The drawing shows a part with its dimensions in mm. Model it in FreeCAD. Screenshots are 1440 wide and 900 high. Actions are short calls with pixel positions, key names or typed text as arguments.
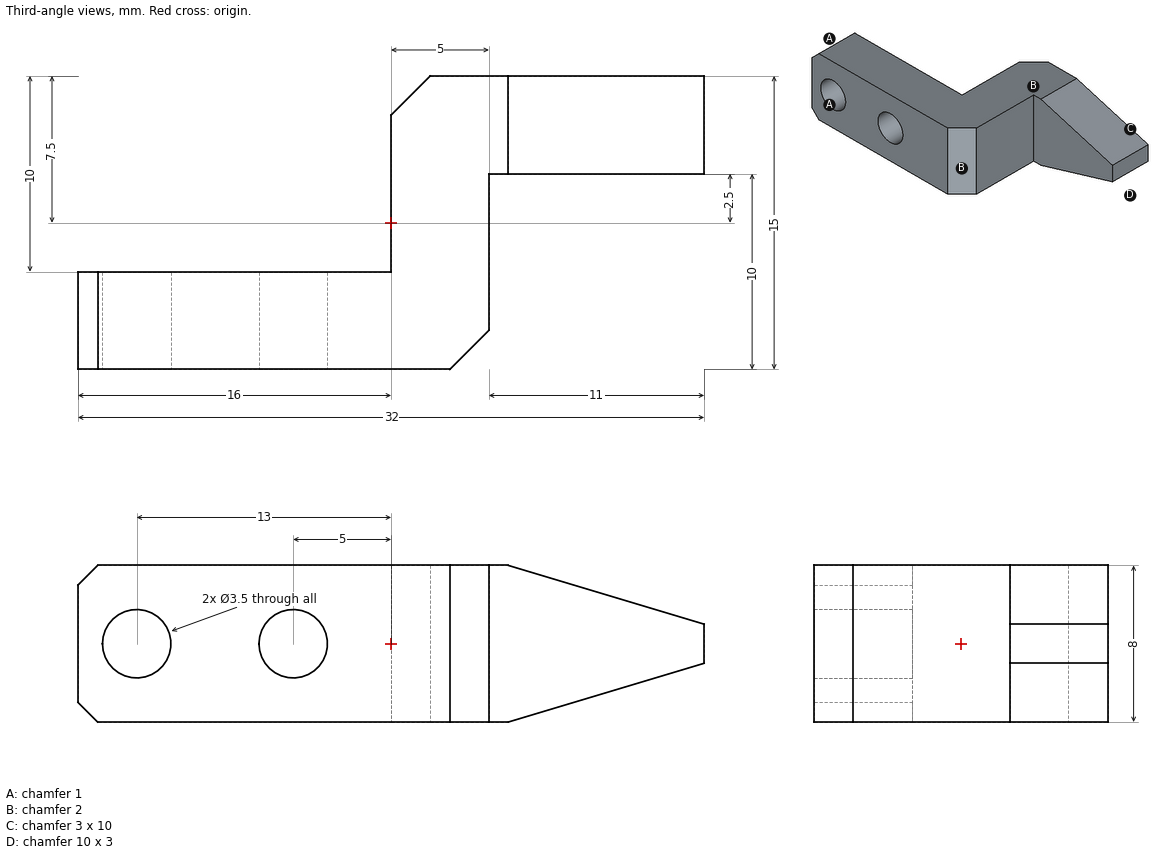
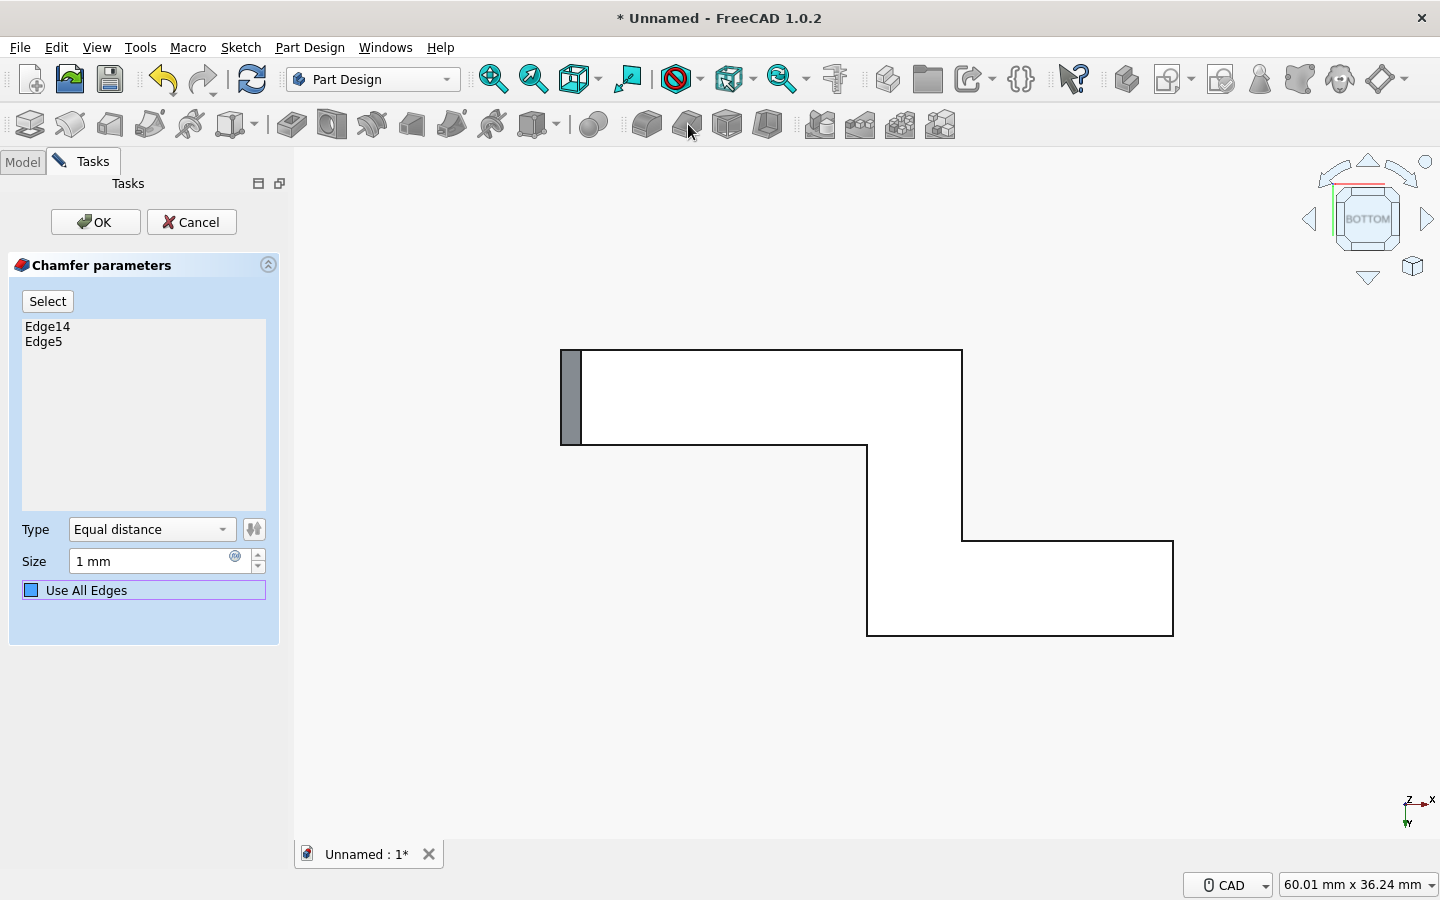
click(96, 222)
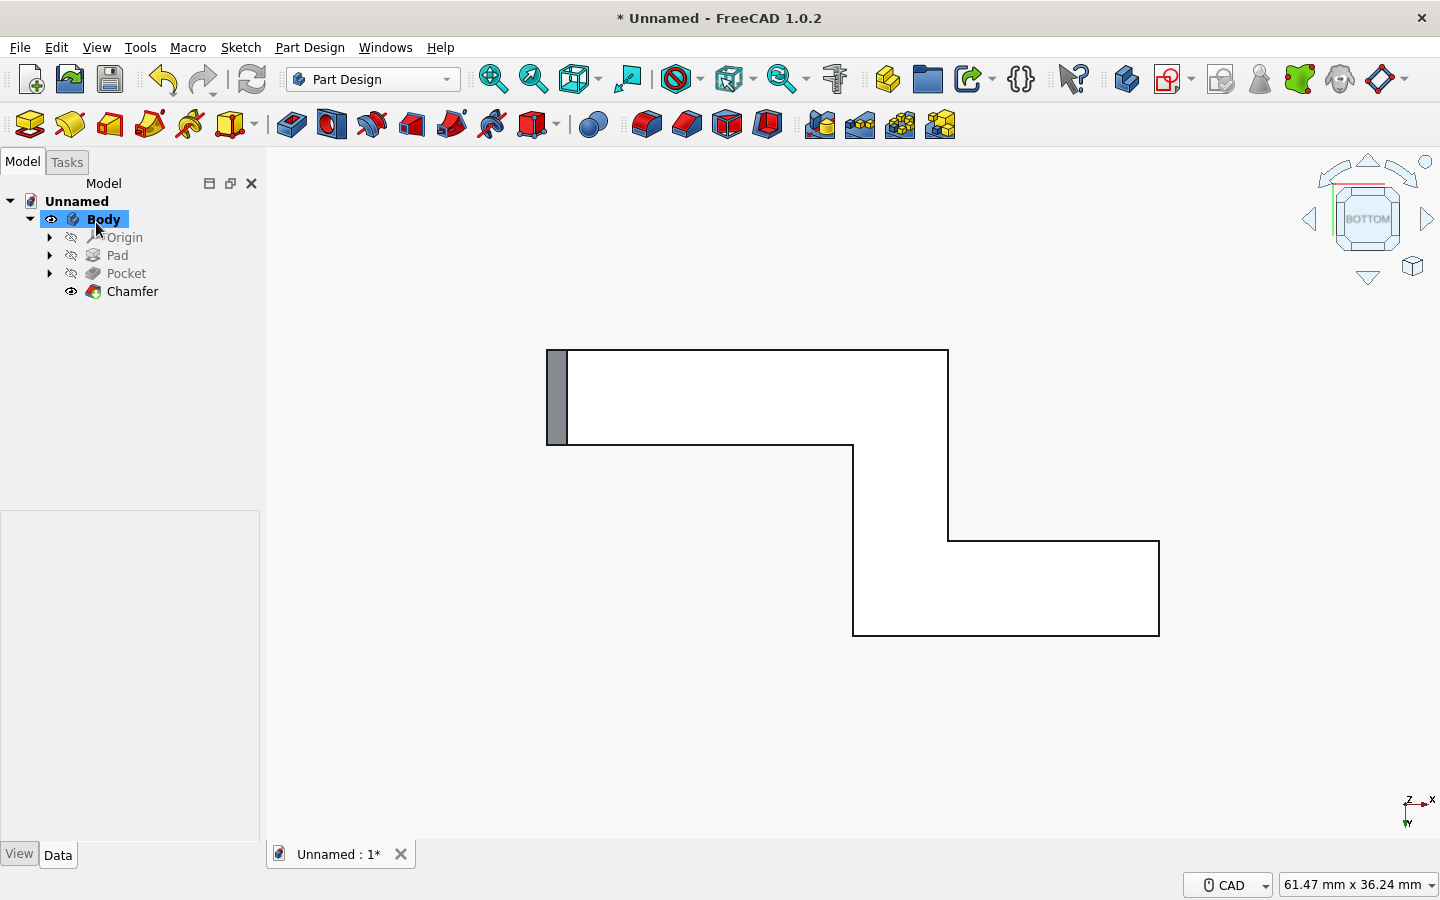
key(0)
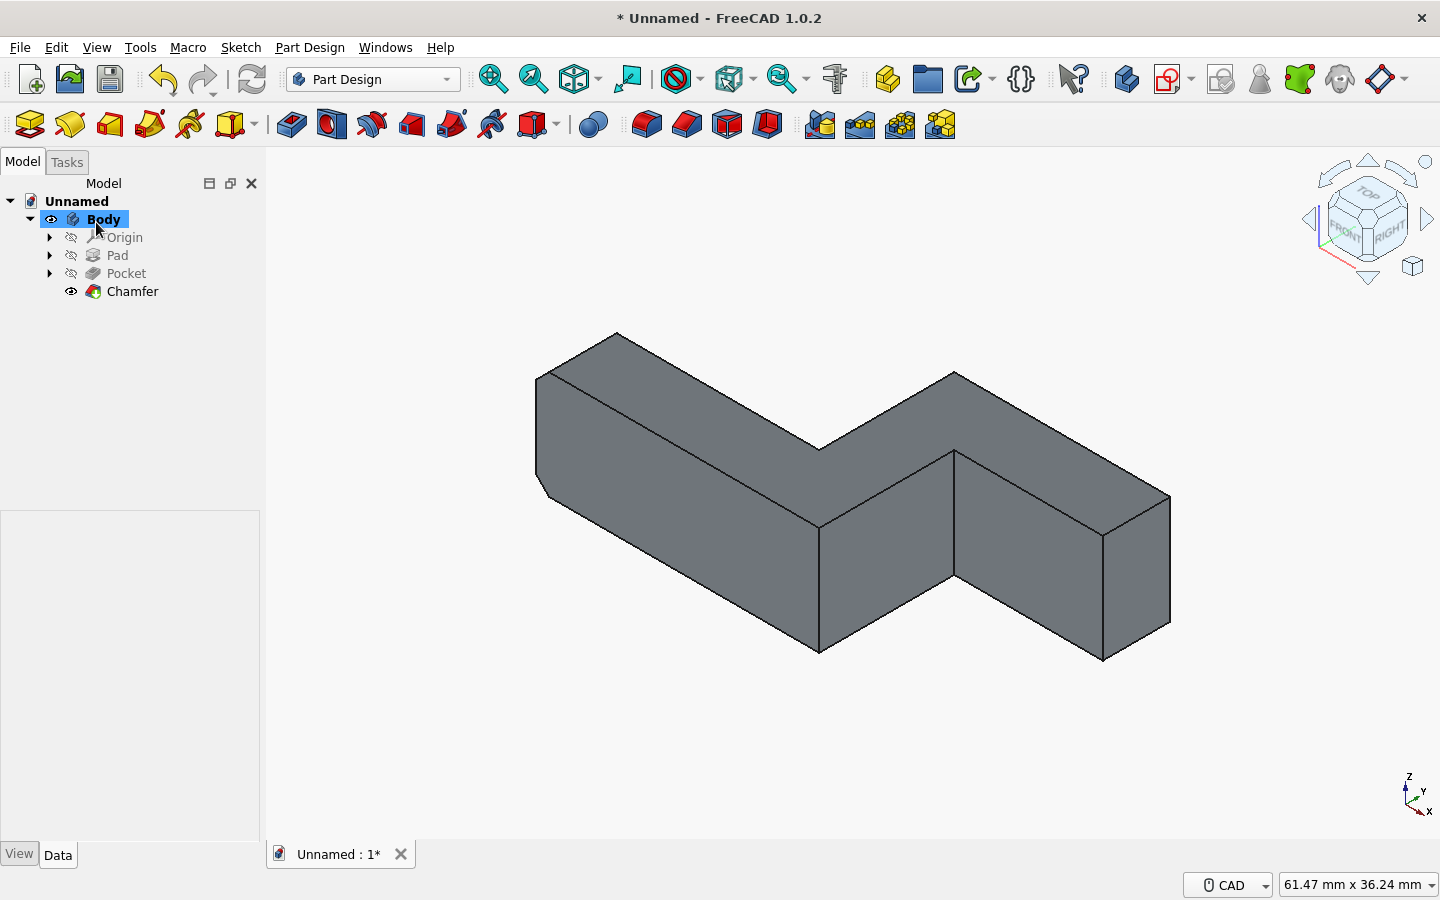
click(819, 589)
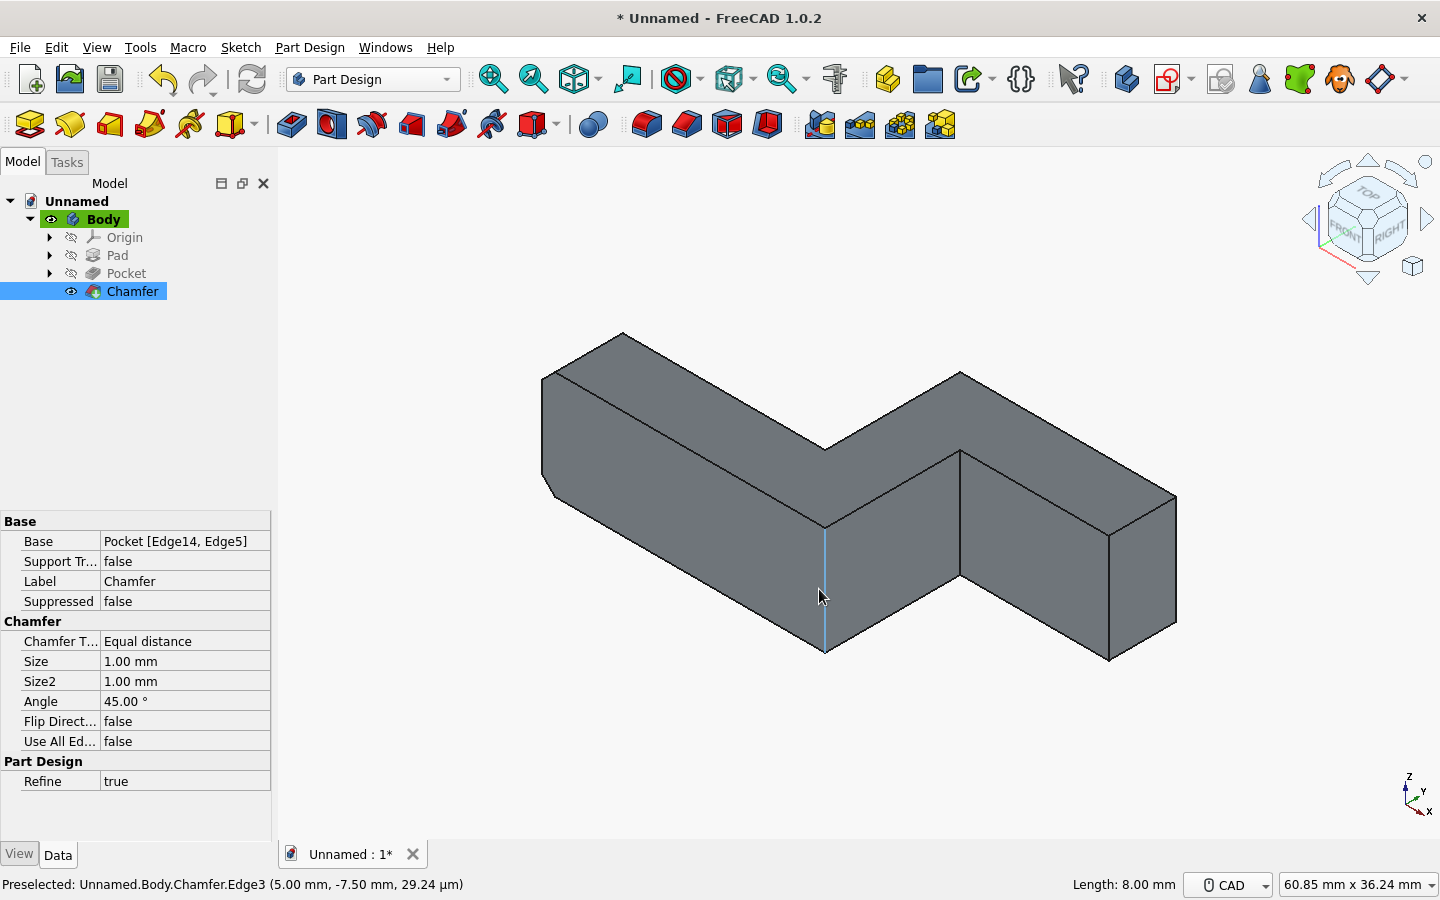
key(2)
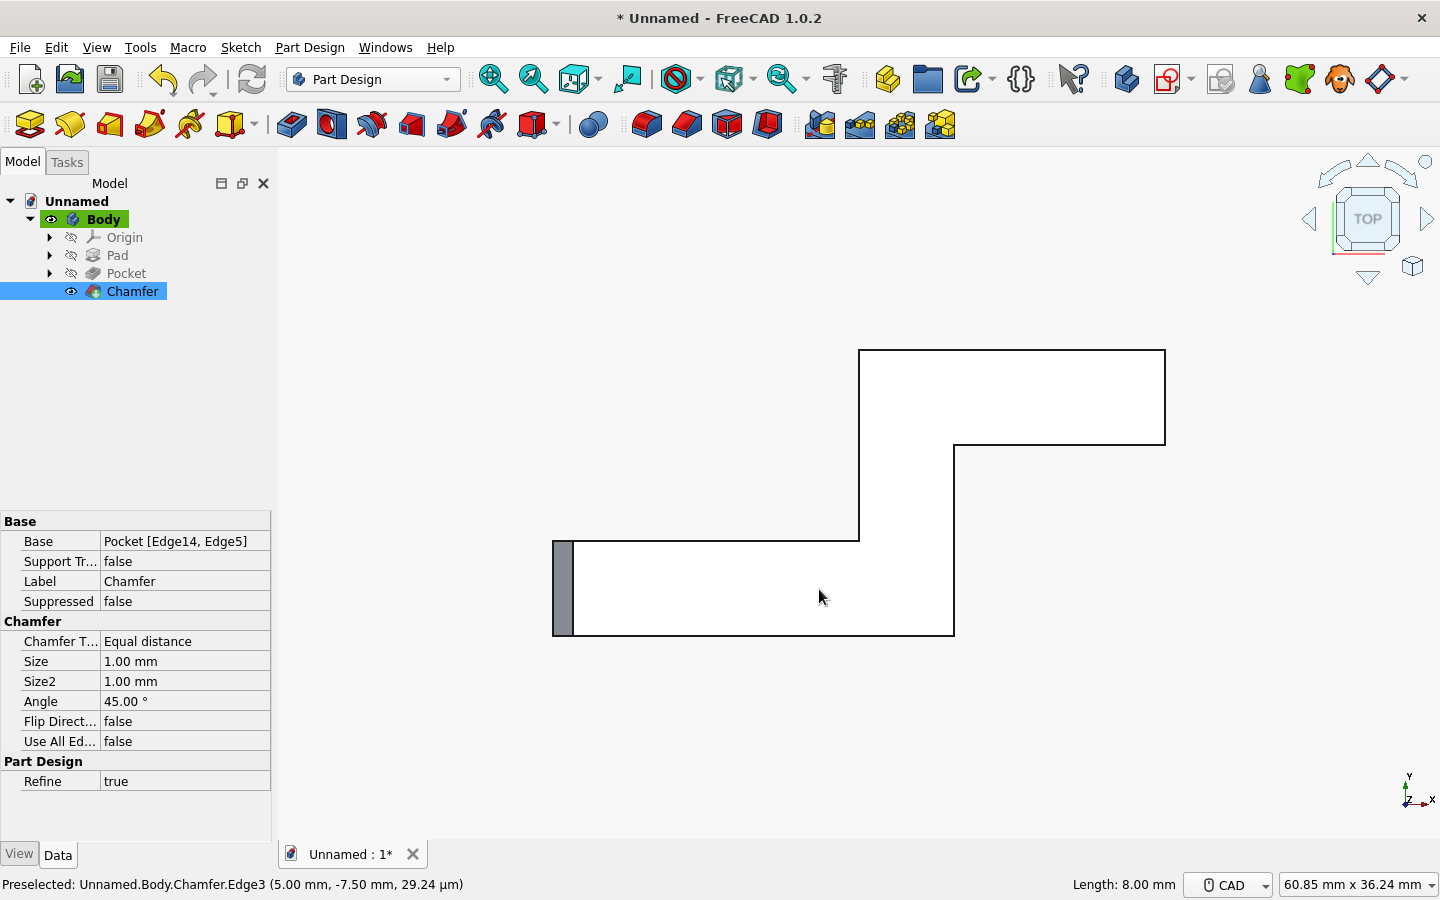
key(1)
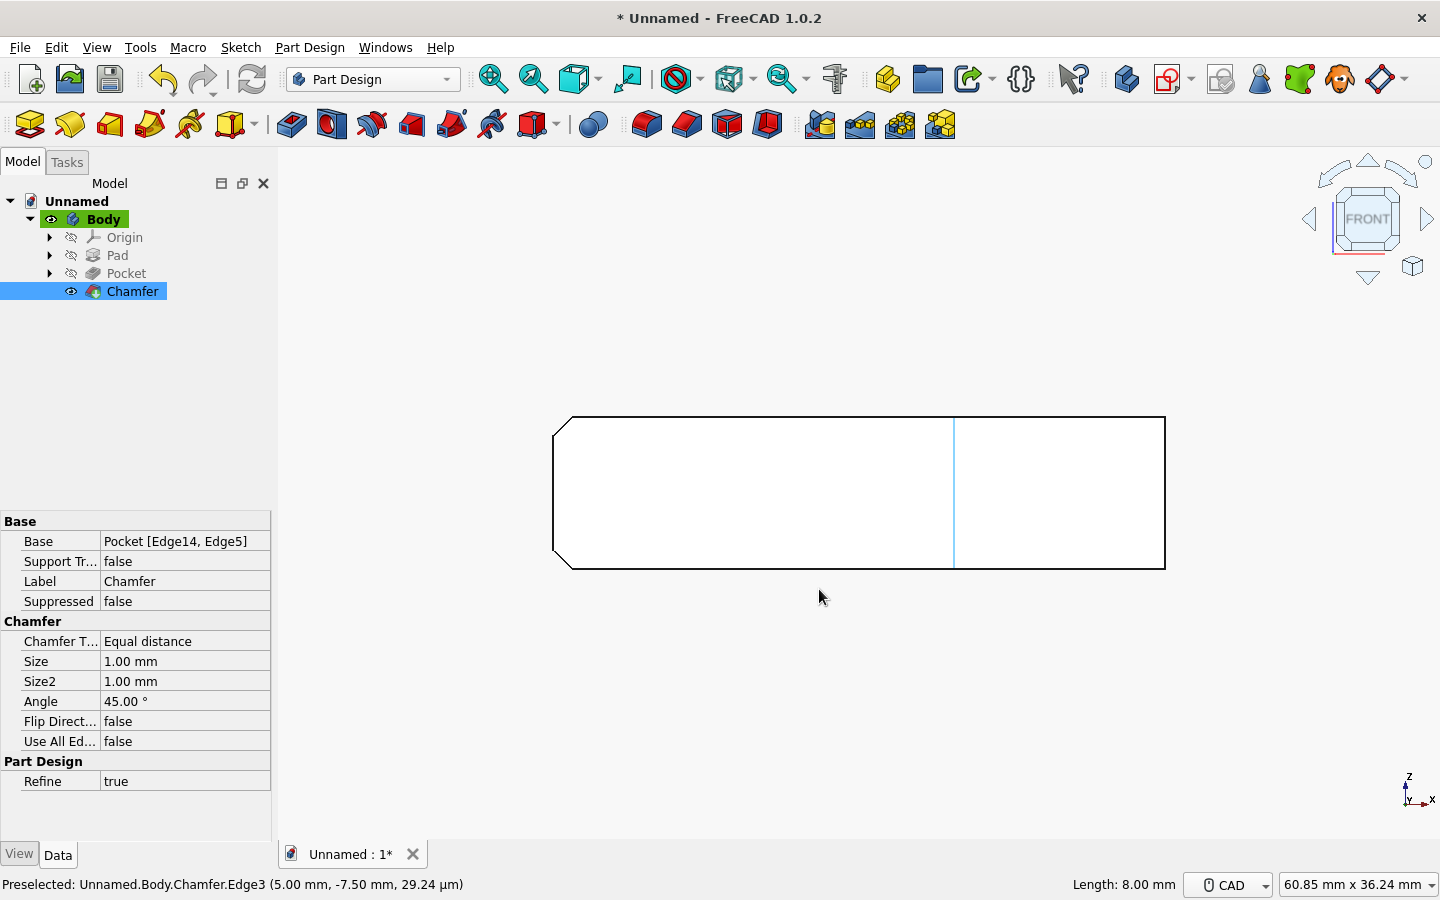
key(3)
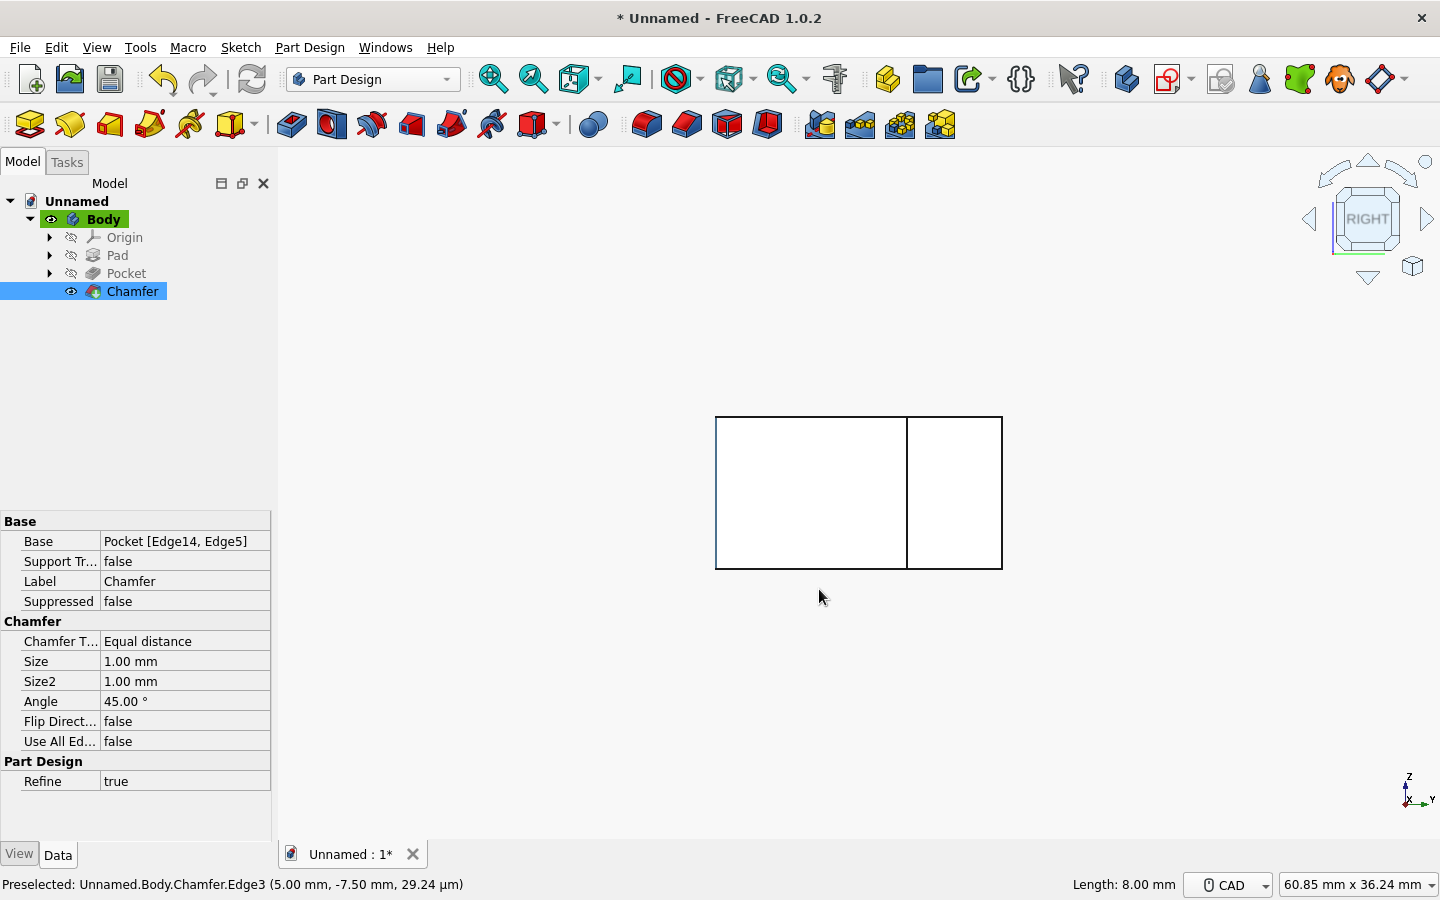
click(494, 80)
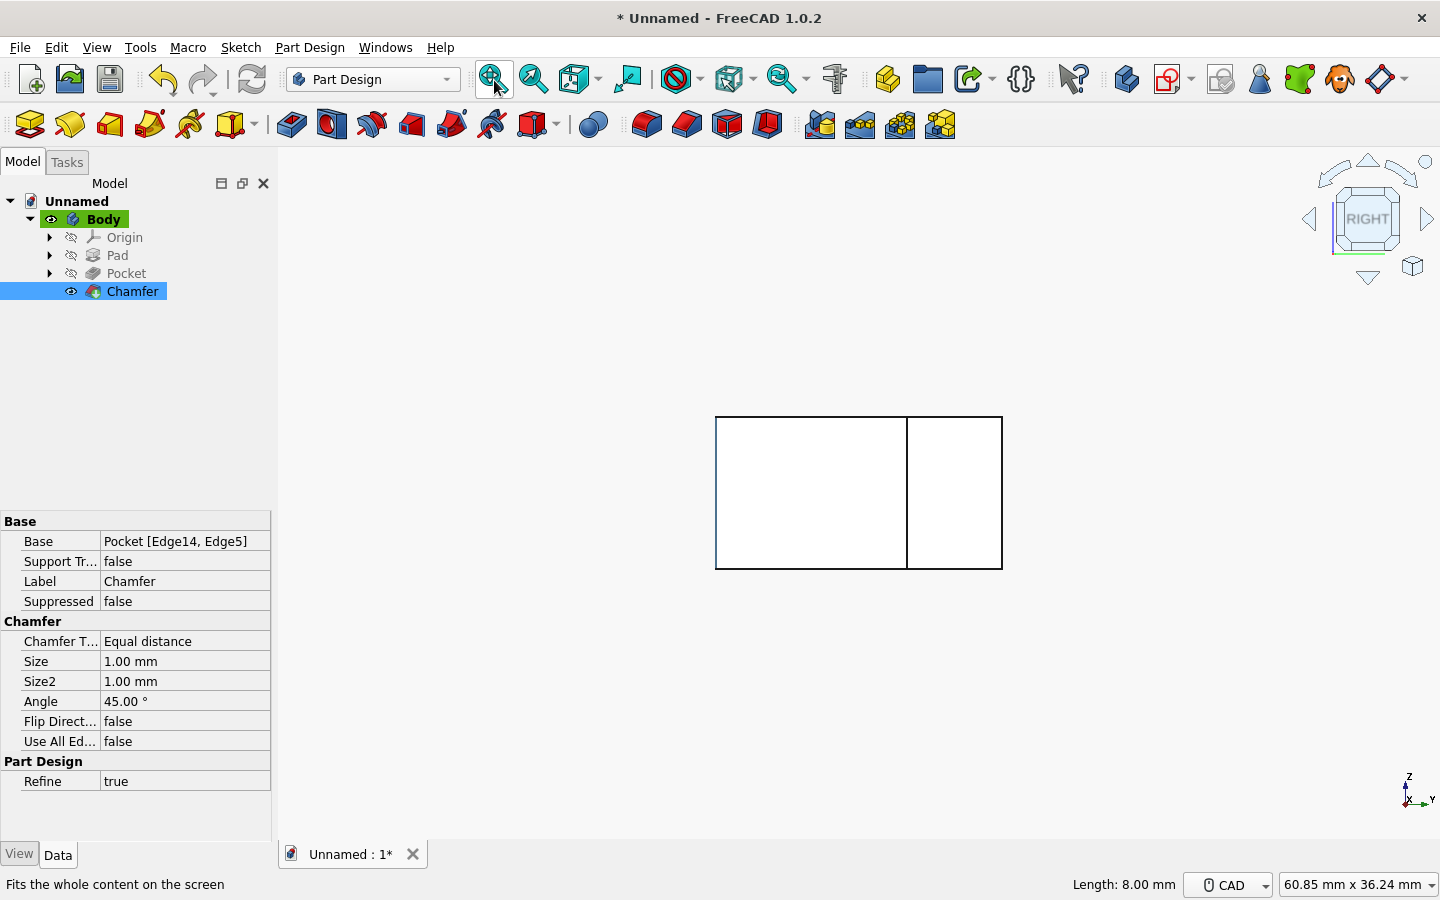
key(5)